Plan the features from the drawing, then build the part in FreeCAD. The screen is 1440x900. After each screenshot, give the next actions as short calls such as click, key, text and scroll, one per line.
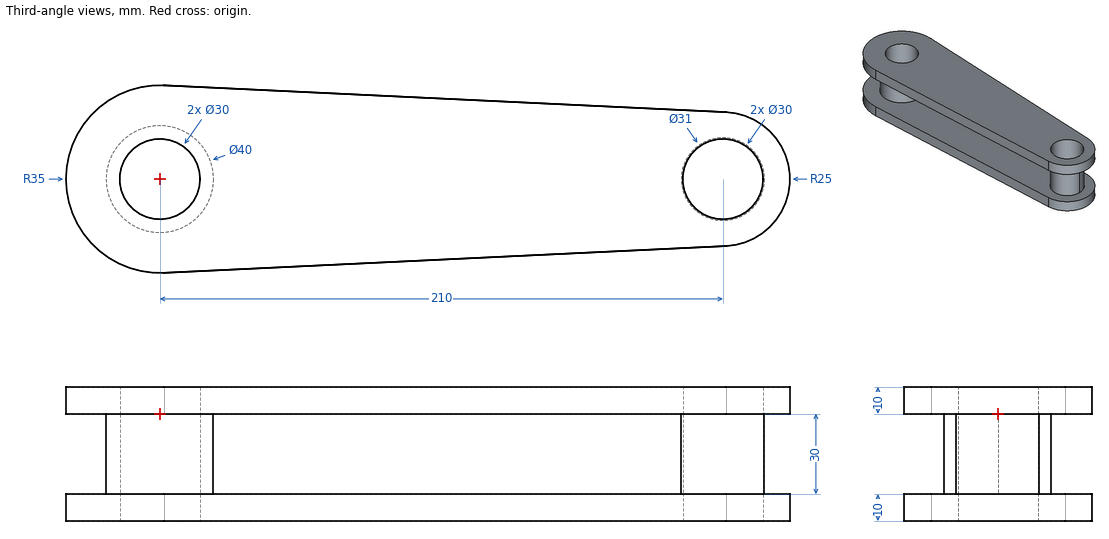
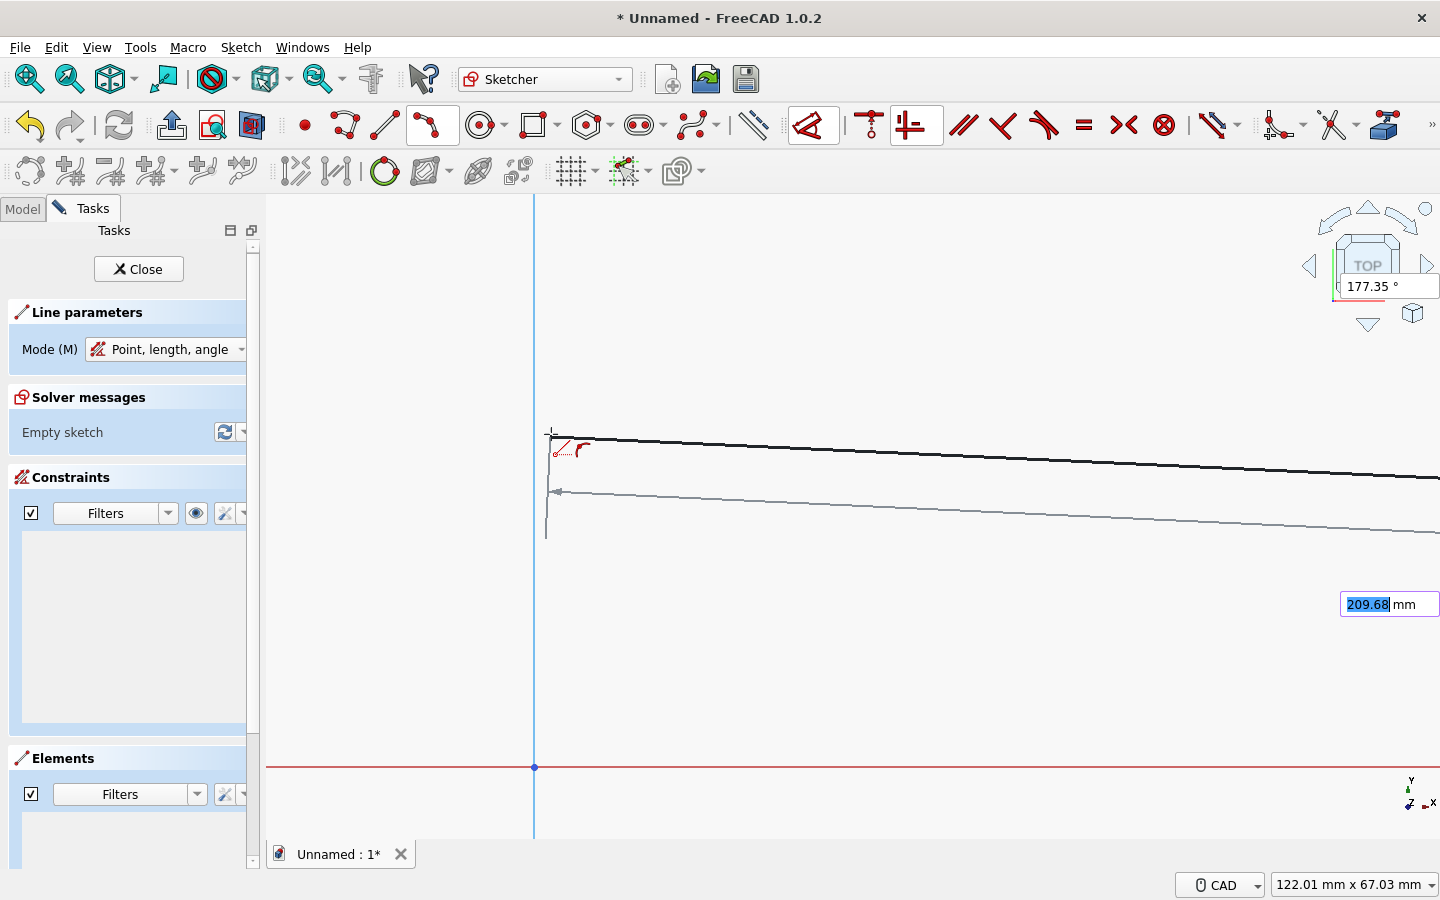
click(551, 431)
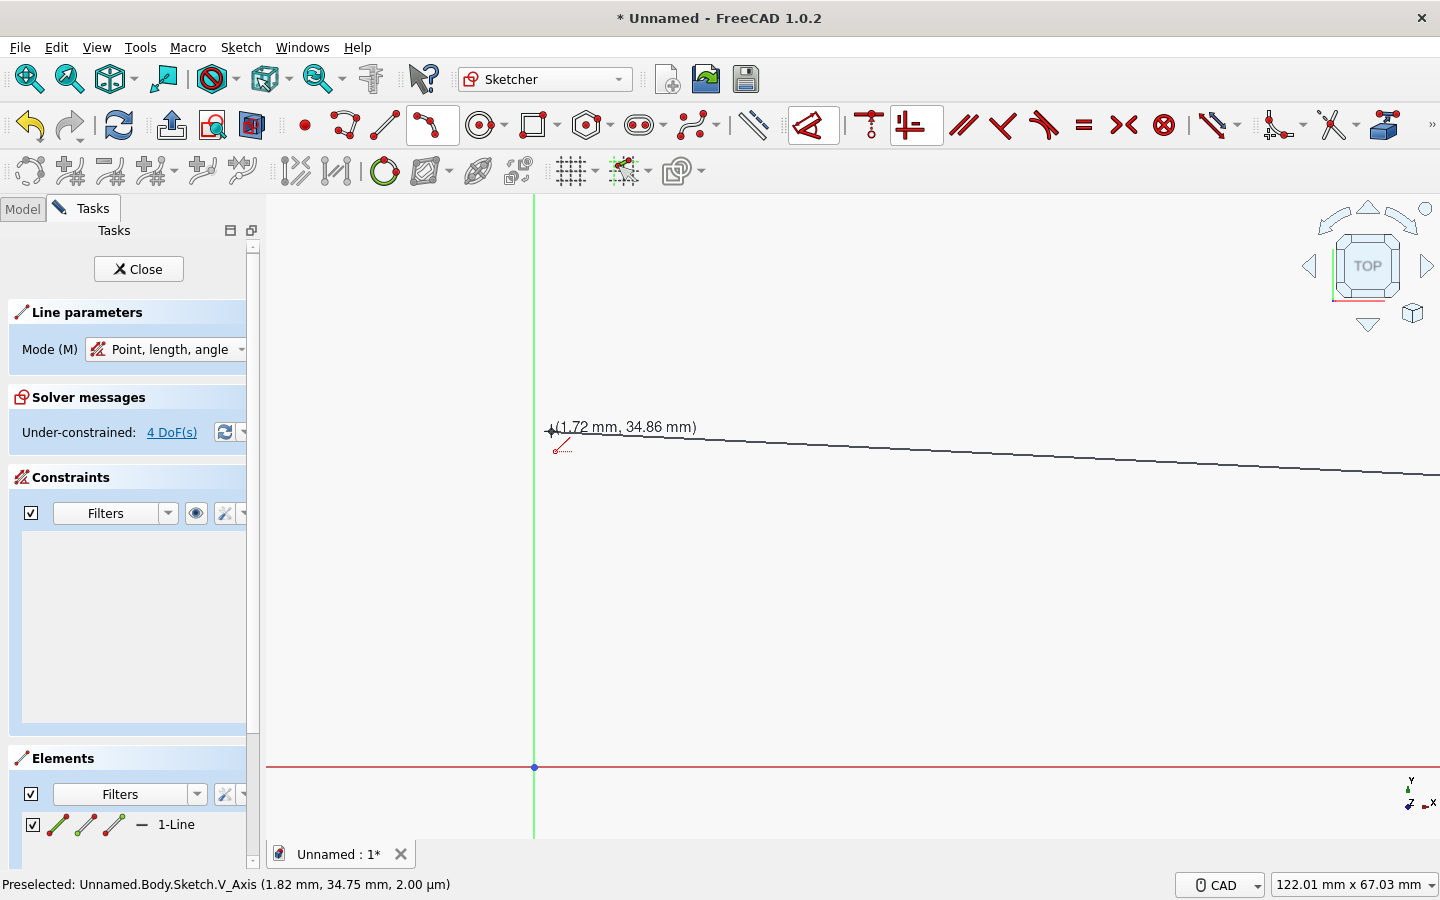
scroll(551, 434, down, 7)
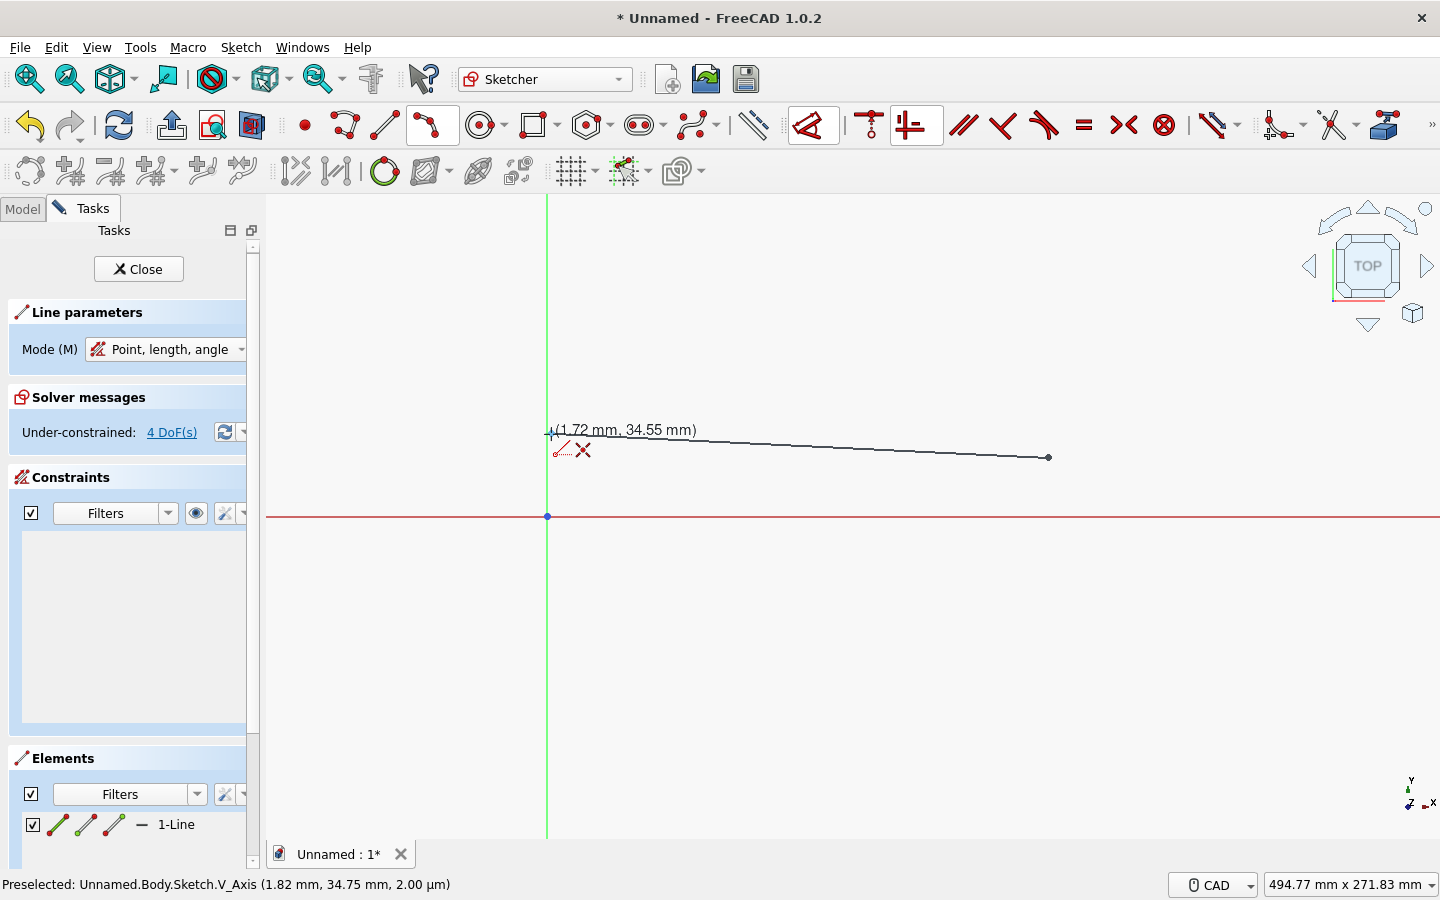
scroll(551, 599, up, 7)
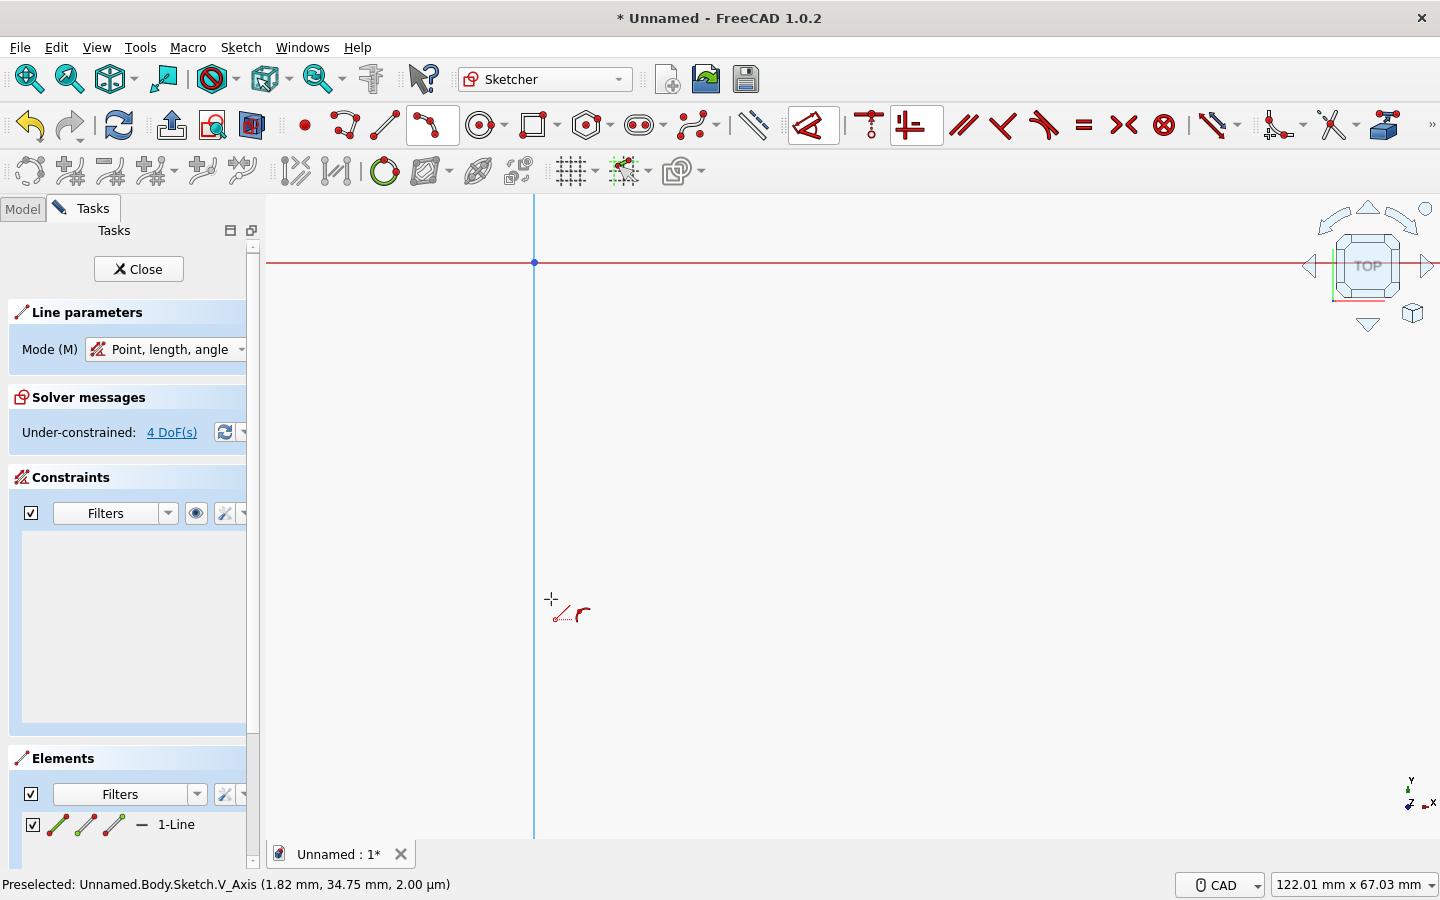
click(551, 599)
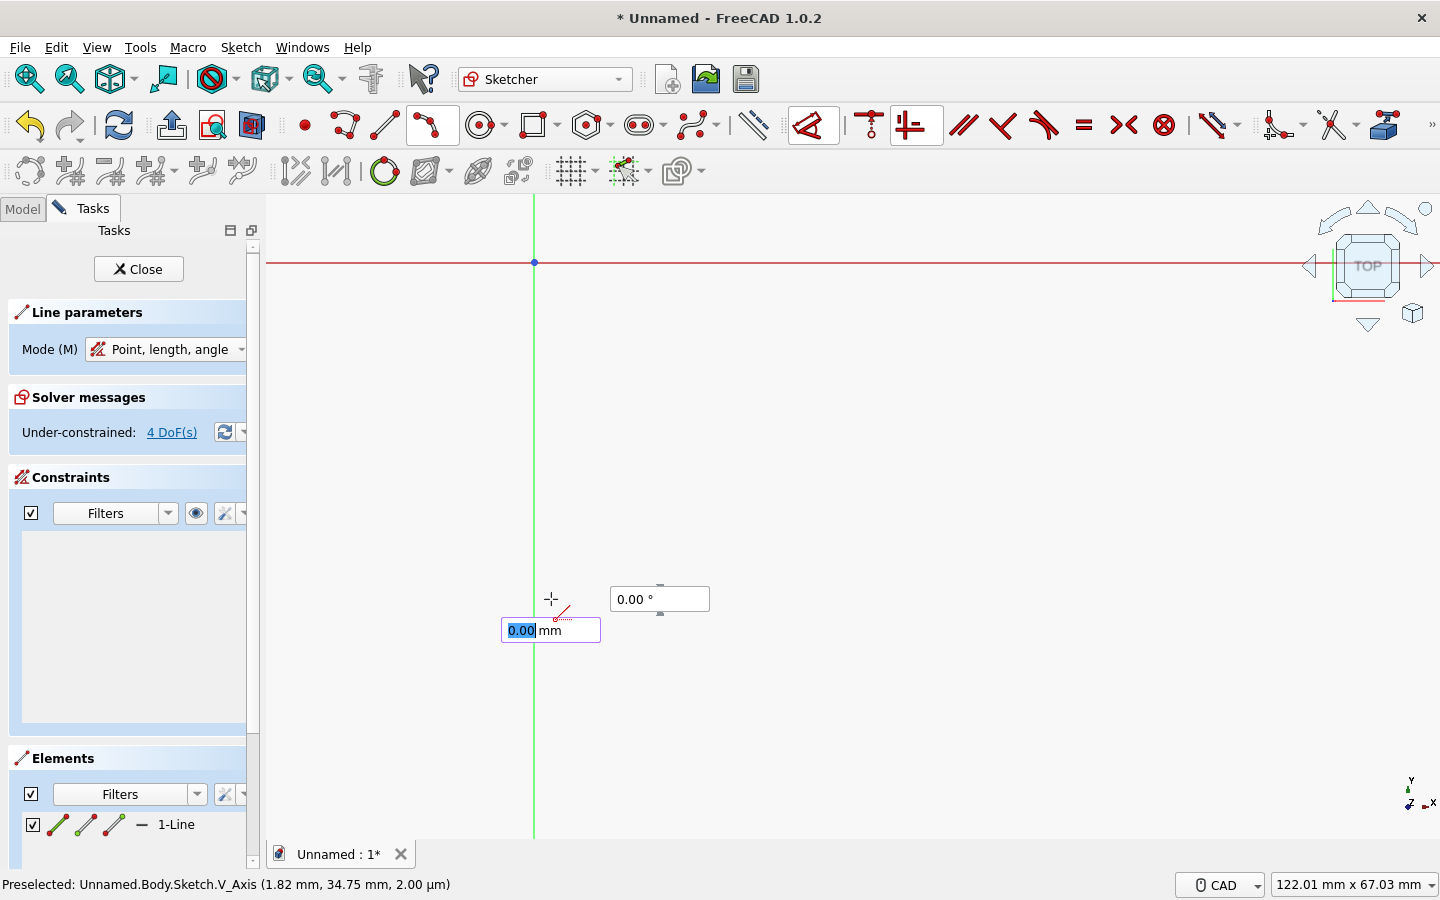
scroll(551, 600, down, 7)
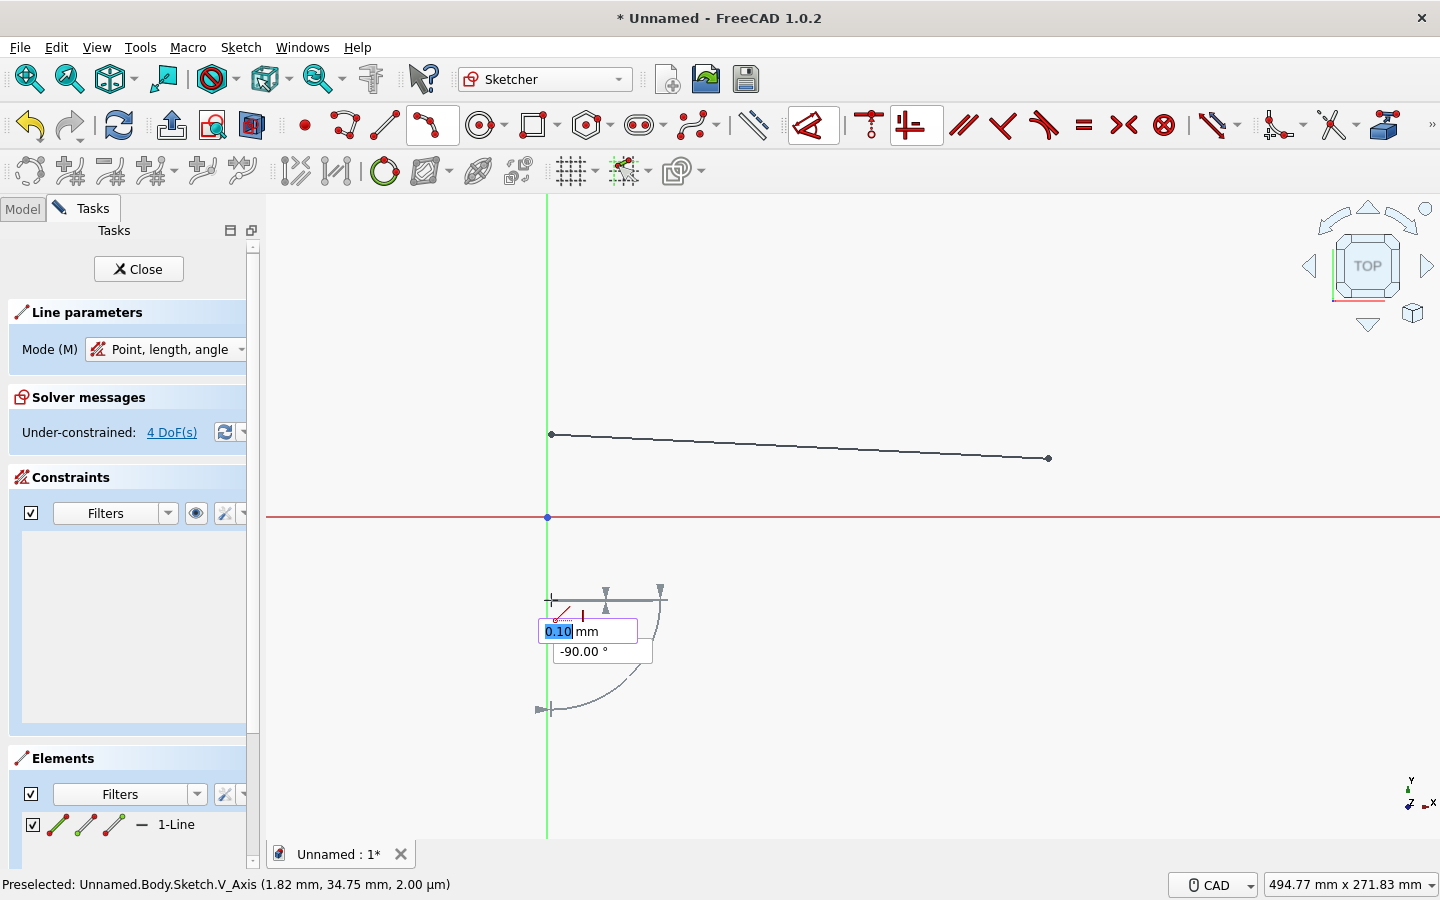
click(1048, 576)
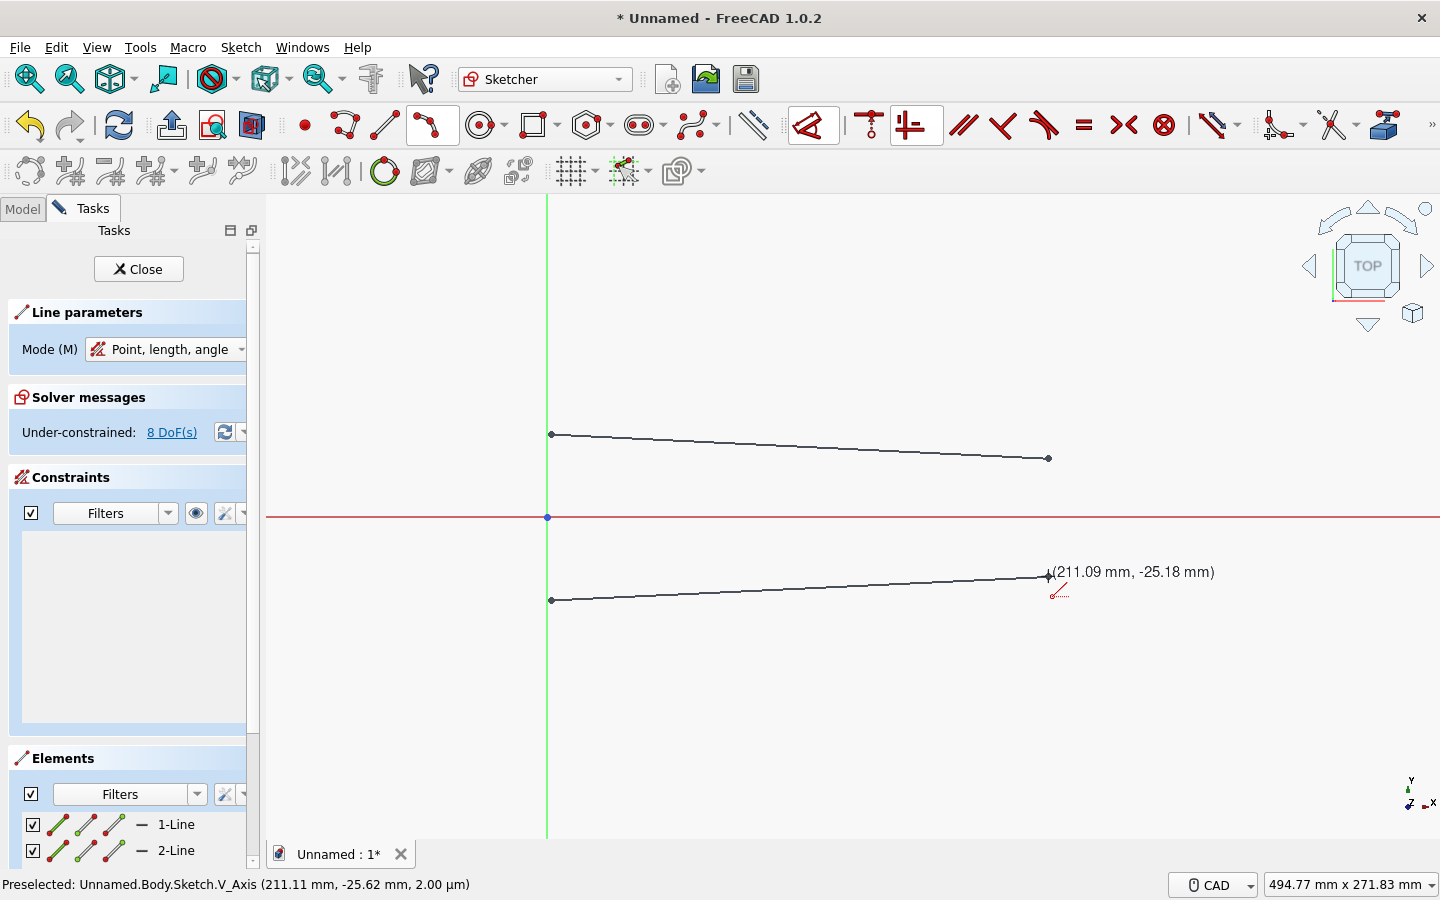
click(426, 126)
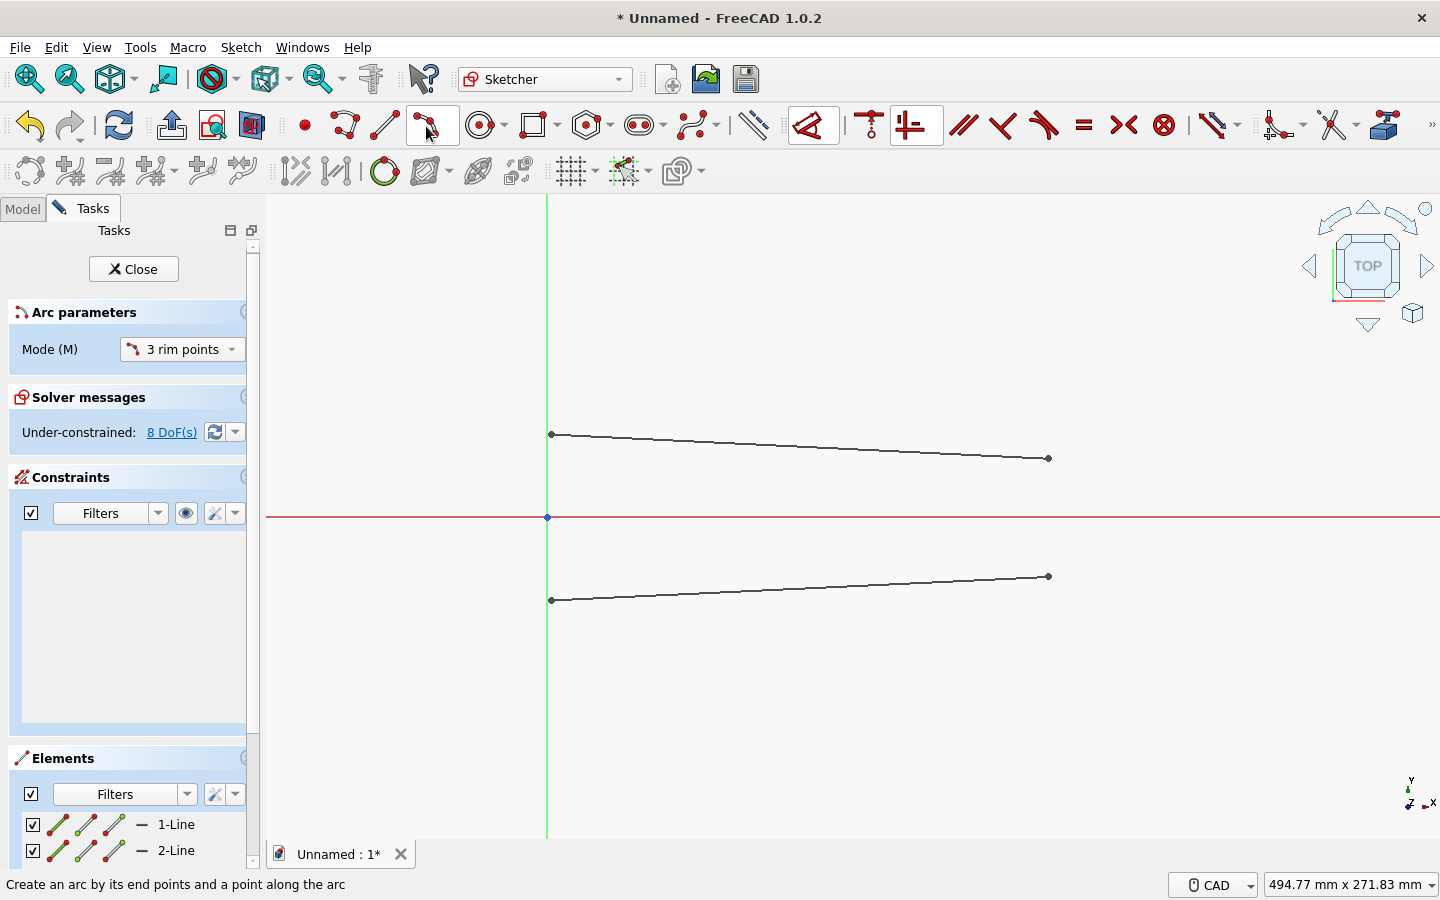
scroll(551, 434, up, 7)